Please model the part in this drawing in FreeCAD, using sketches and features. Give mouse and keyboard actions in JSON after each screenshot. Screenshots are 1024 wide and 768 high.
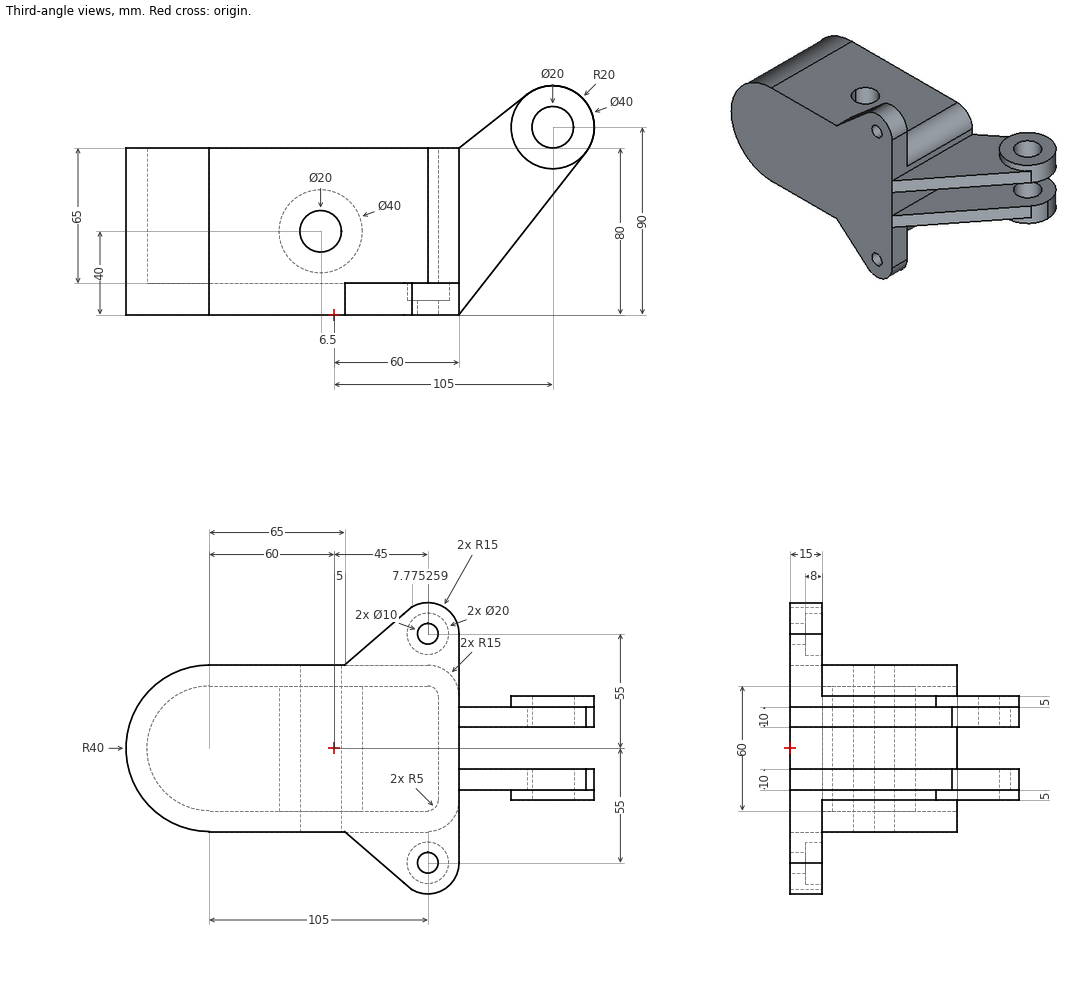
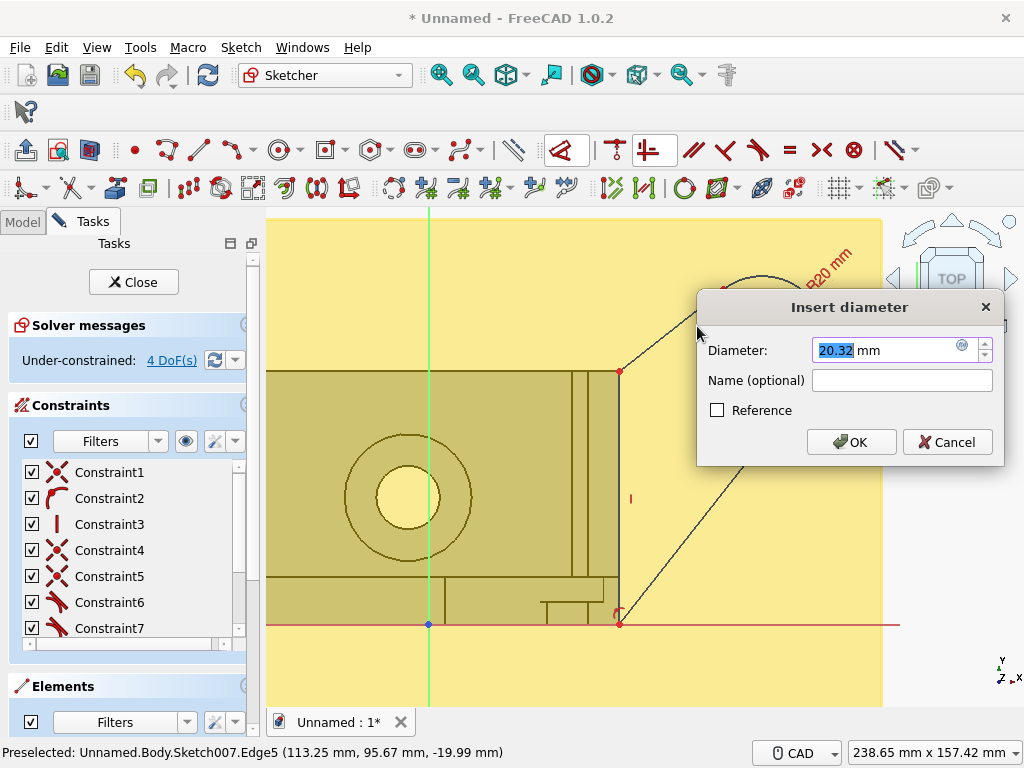
{"action": "type", "text": "20"}
{"action": "key", "text": "Return"}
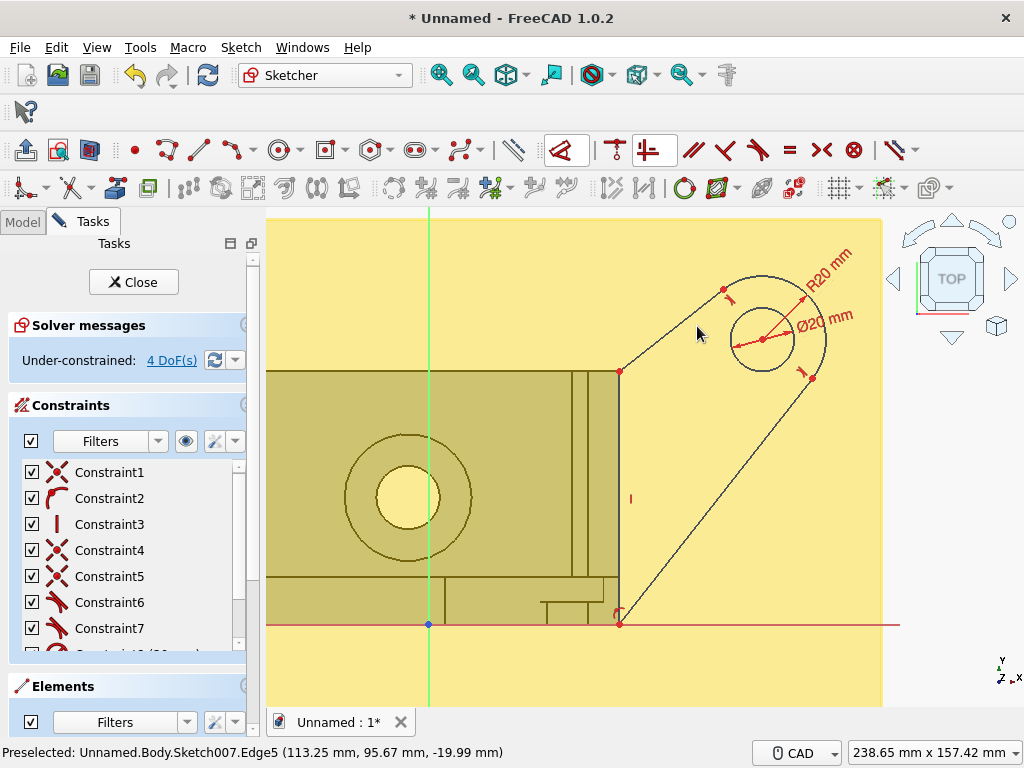
{"action": "left_click", "coordinate": [619, 448]}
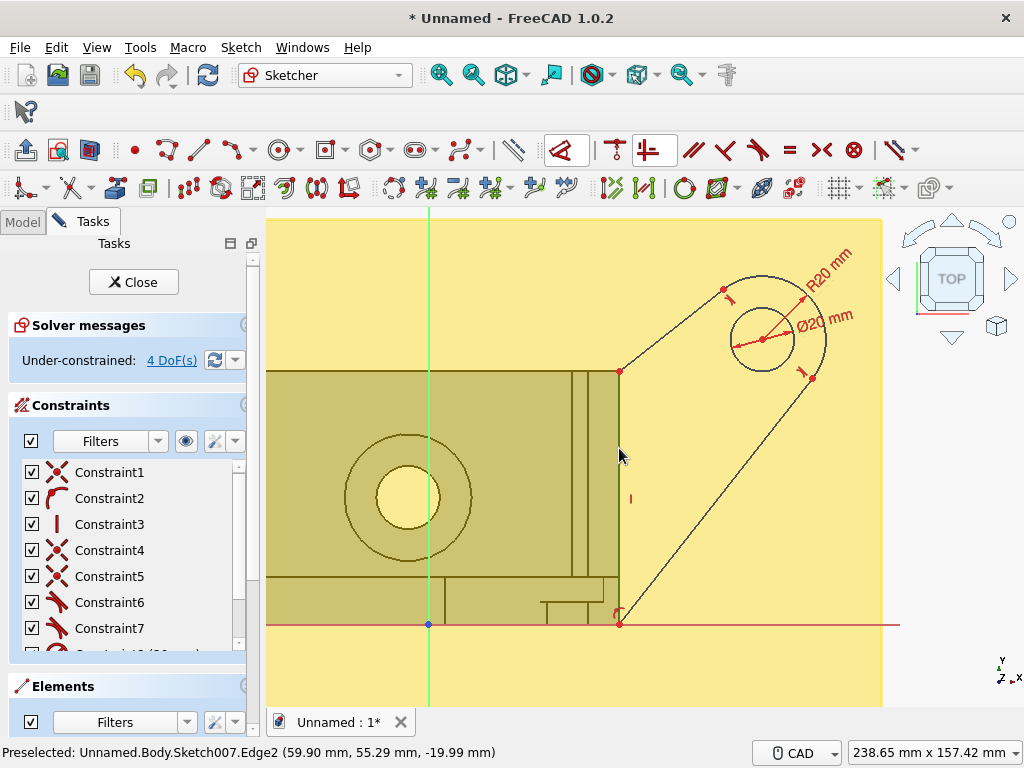
{"action": "left_click", "coordinate": [584, 150]}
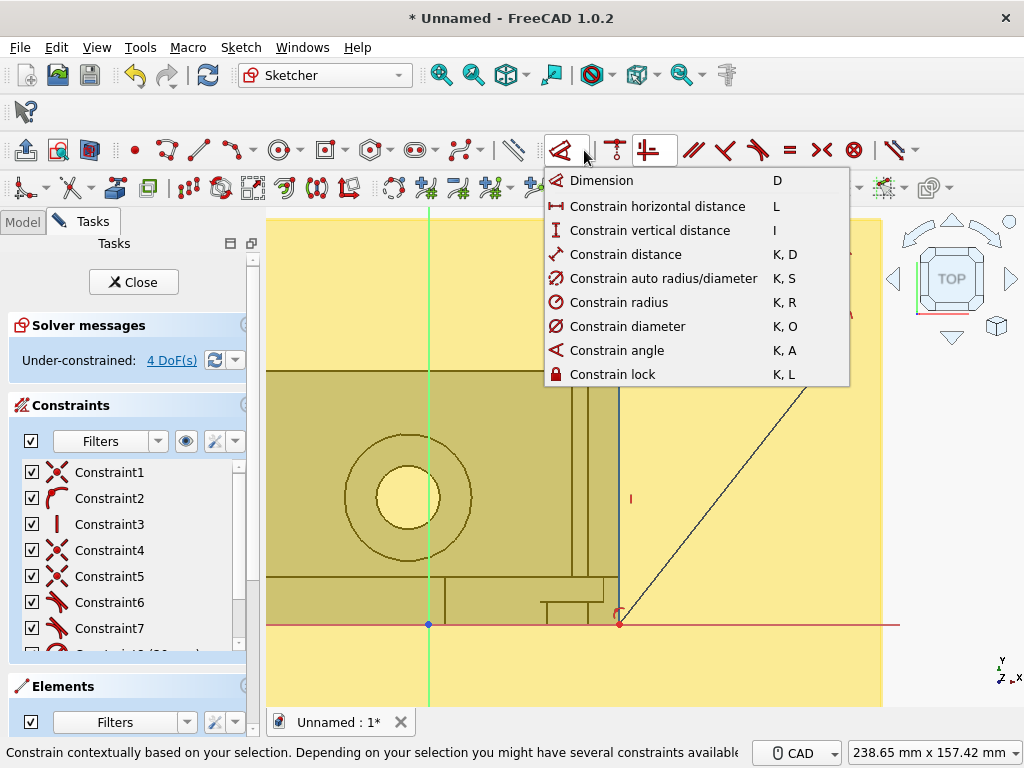
{"action": "left_click", "coordinate": [697, 230]}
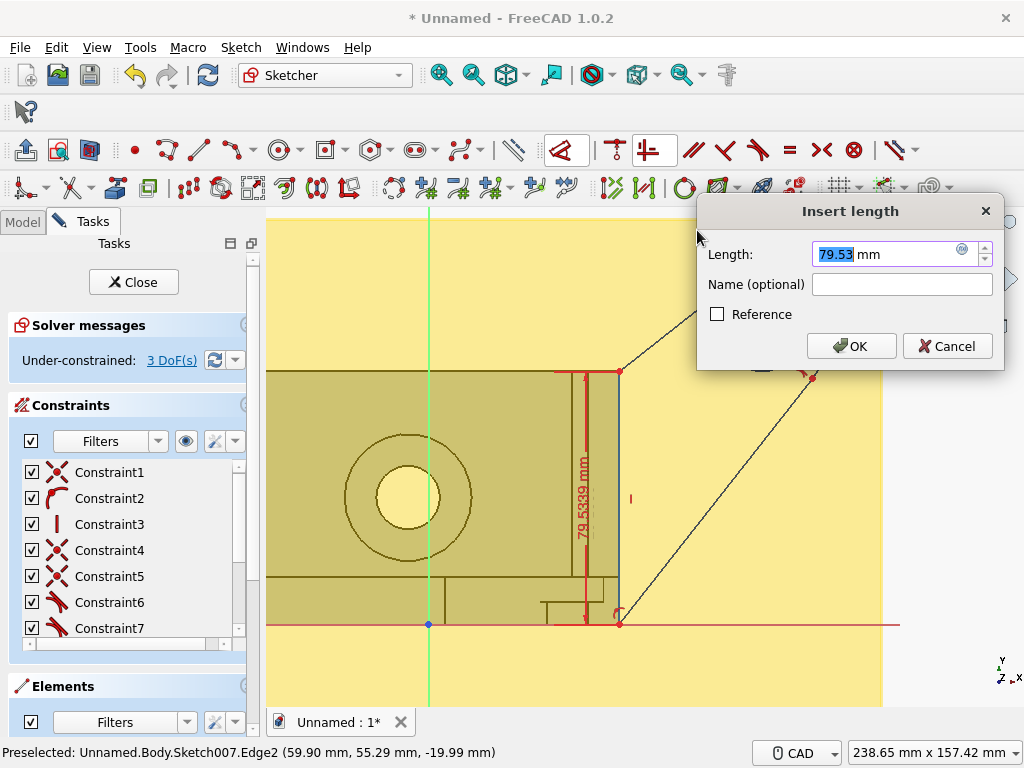
{"action": "type", "text": "80"}
{"action": "key", "text": "Return"}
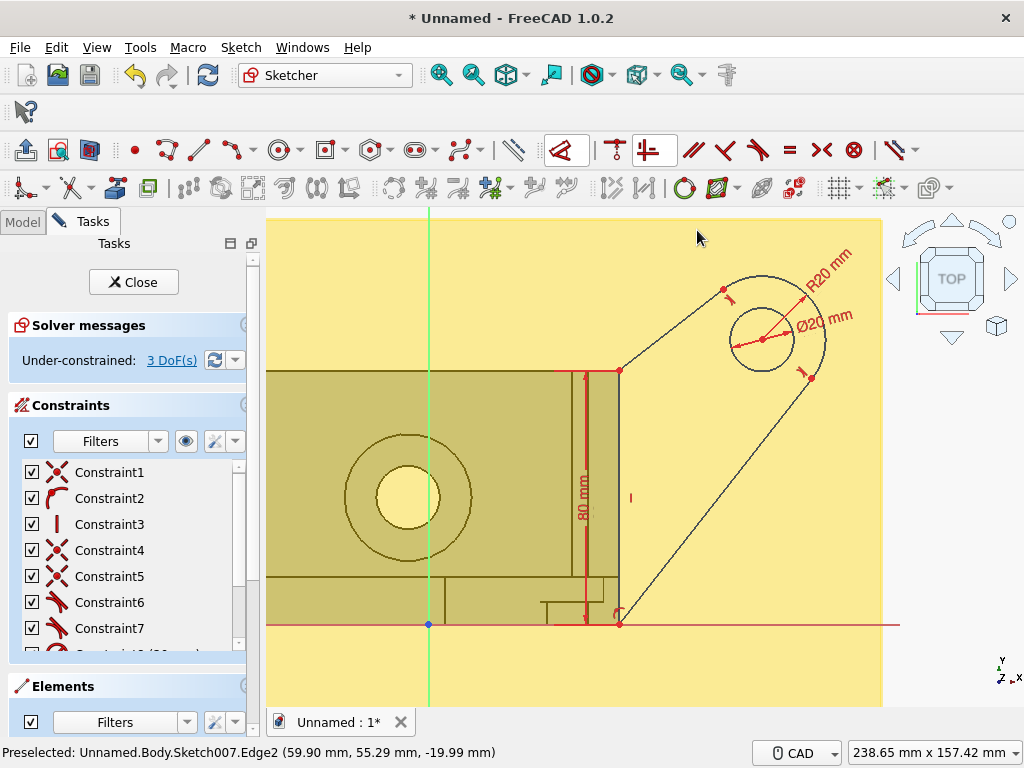
{"action": "left_click", "coordinate": [762, 340]}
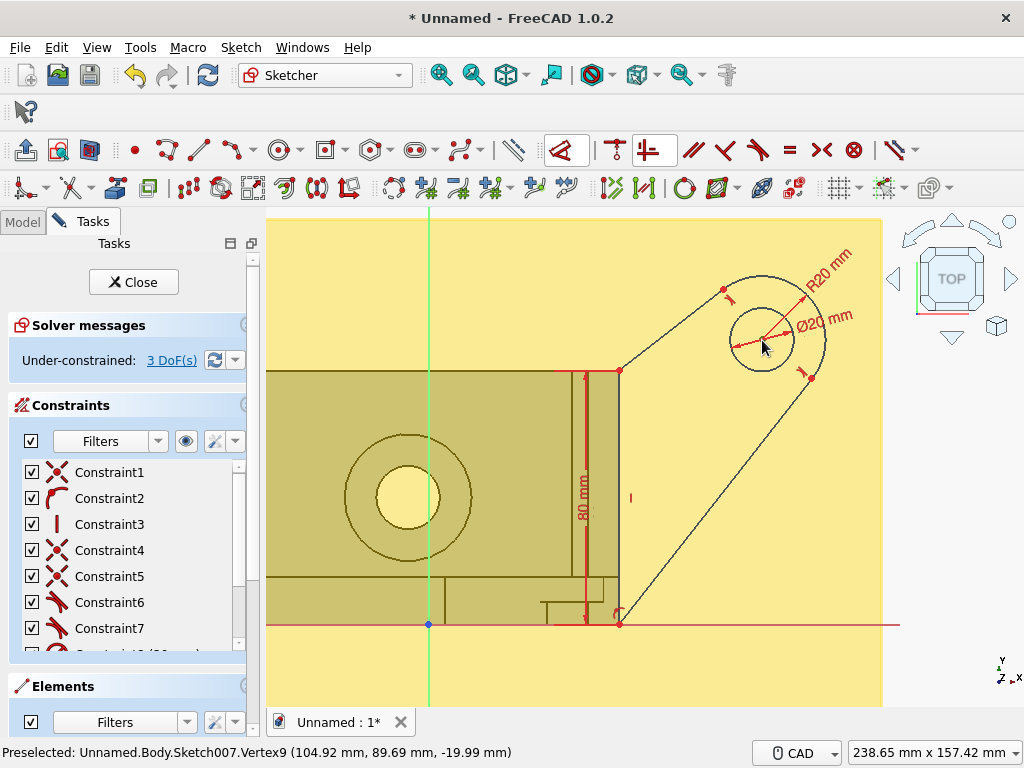
{"action": "left_click", "coordinate": [584, 150]}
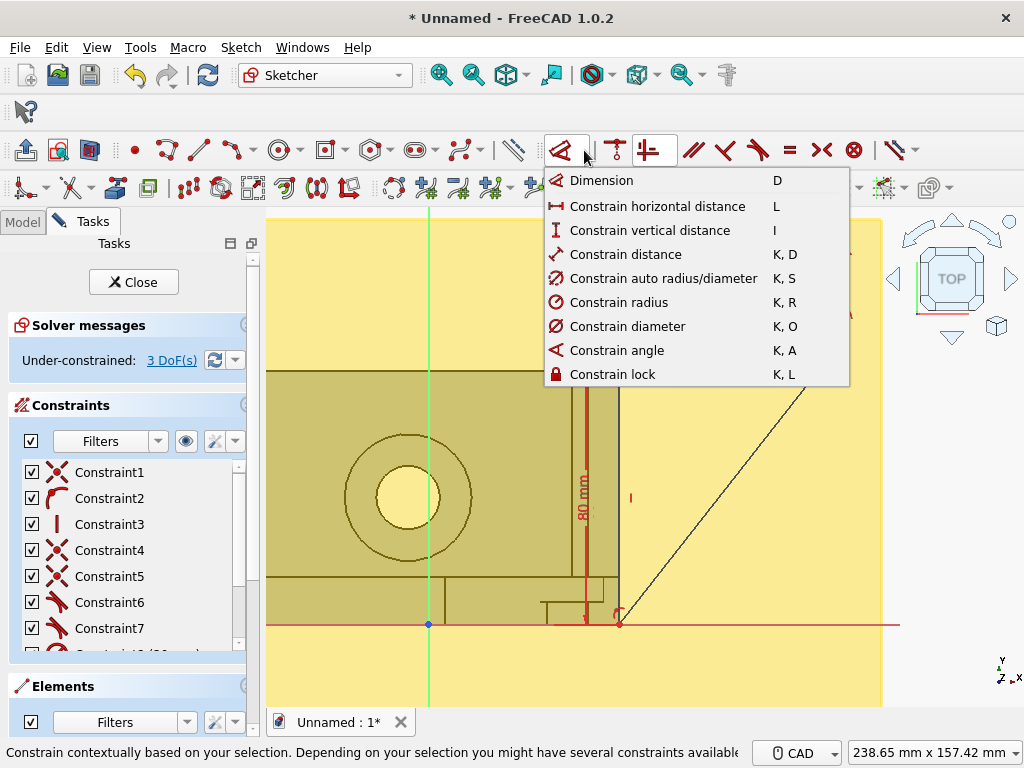
{"action": "left_click", "coordinate": [697, 230]}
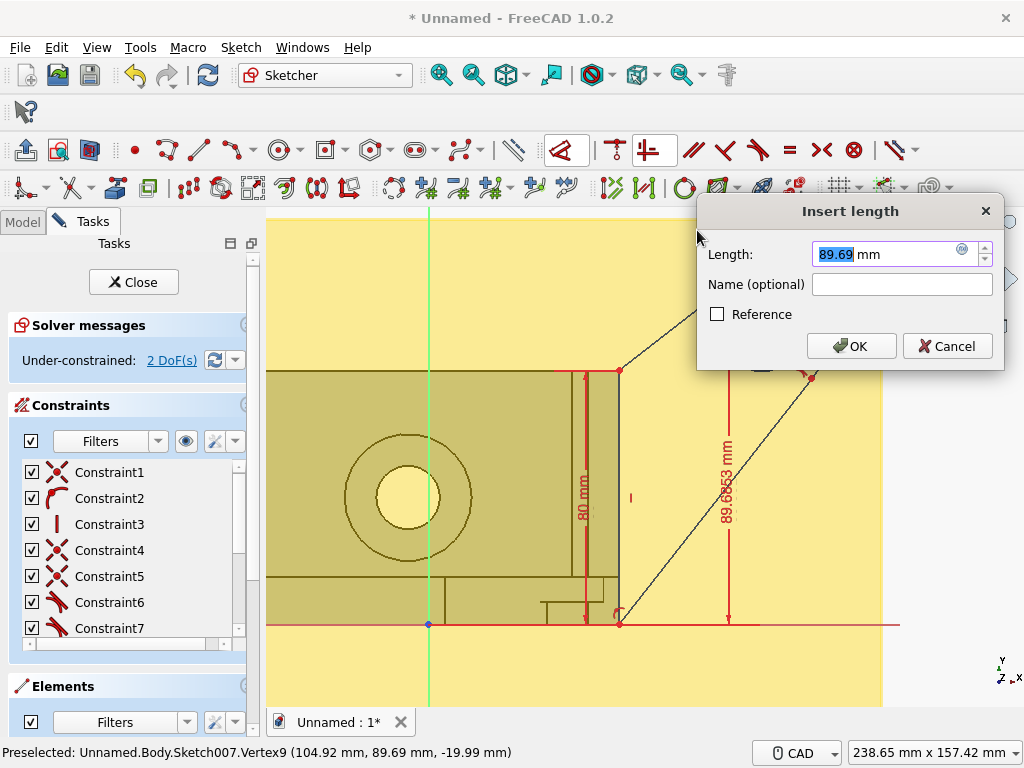
{"action": "type", "text": "90"}
{"action": "key", "text": "Return"}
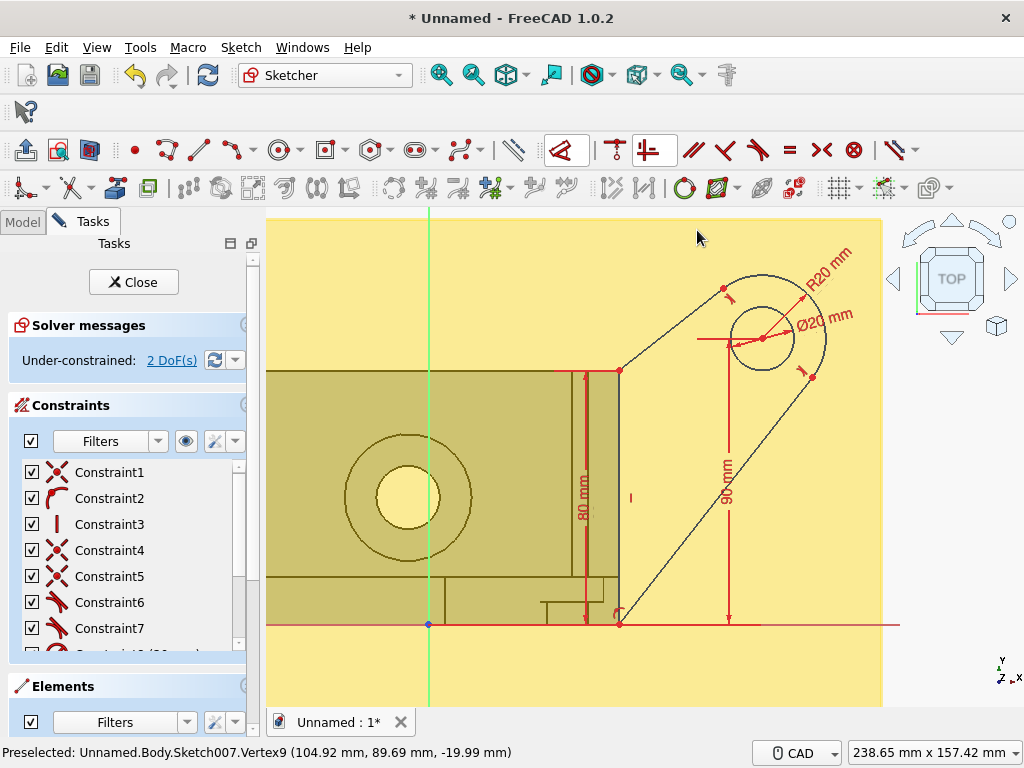
{"action": "left_click", "coordinate": [619, 371]}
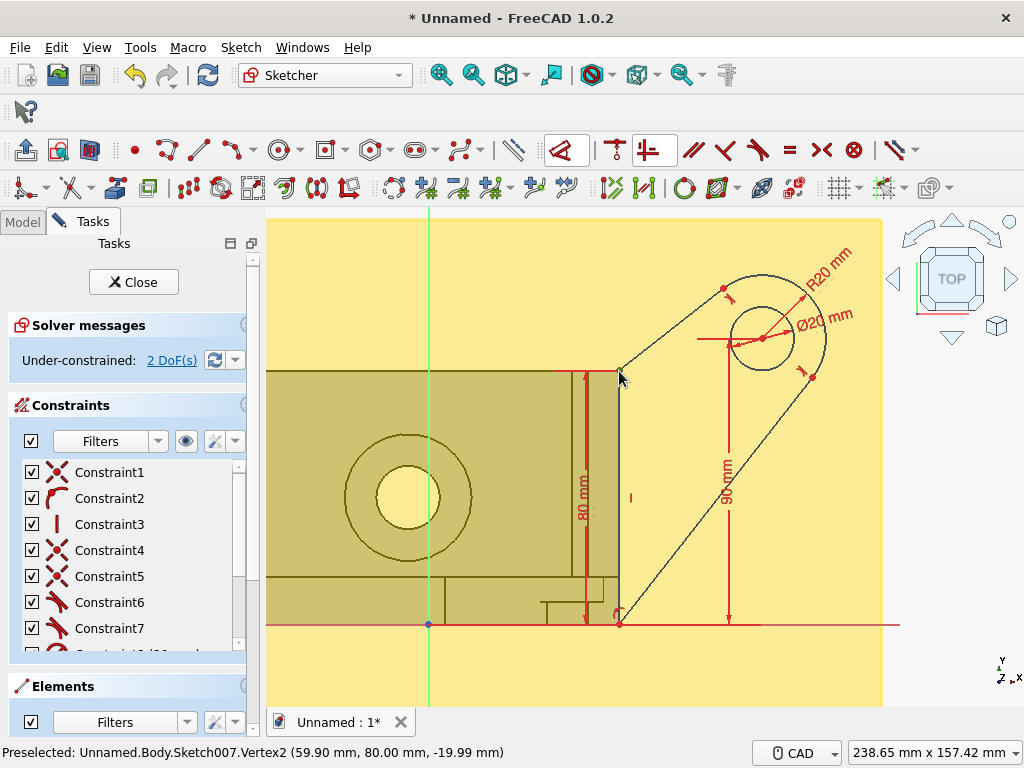
{"action": "left_click", "coordinate": [584, 150]}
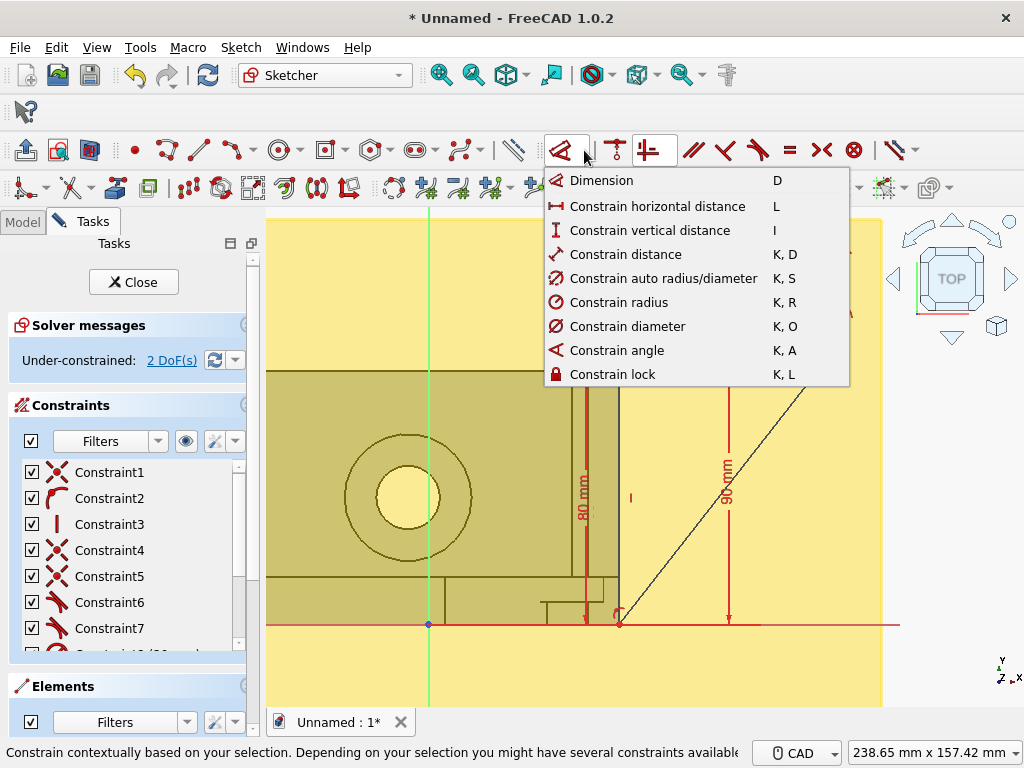
{"action": "left_click", "coordinate": [697, 206]}